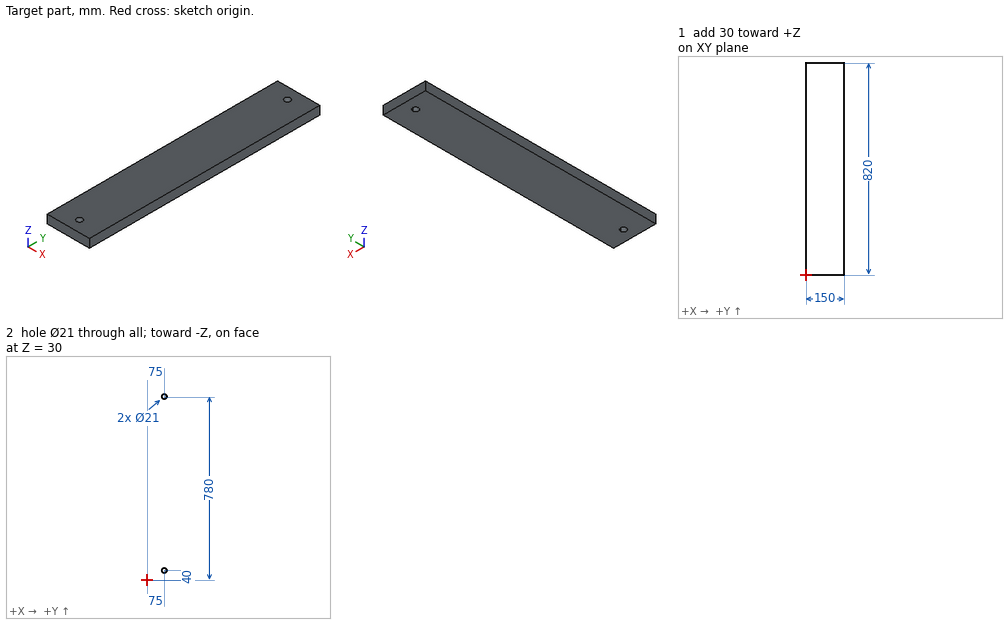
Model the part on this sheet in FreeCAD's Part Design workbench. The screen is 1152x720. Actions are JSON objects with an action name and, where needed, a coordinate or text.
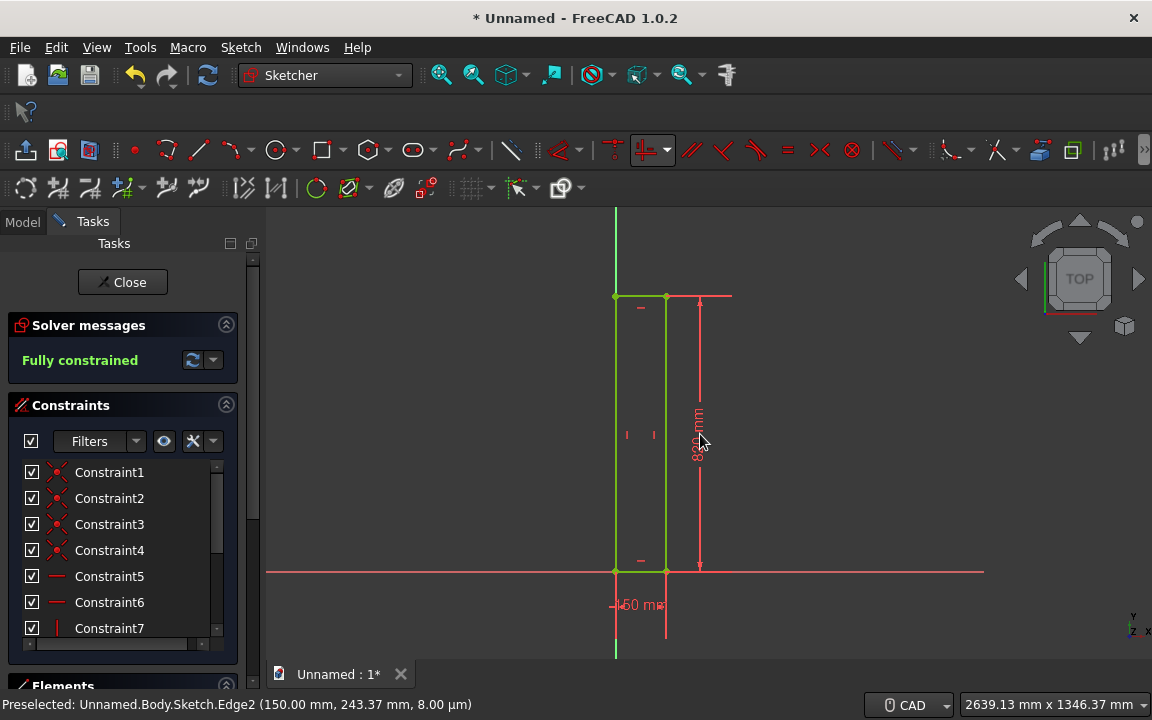
{"action": "left_click", "coordinate": [123, 282]}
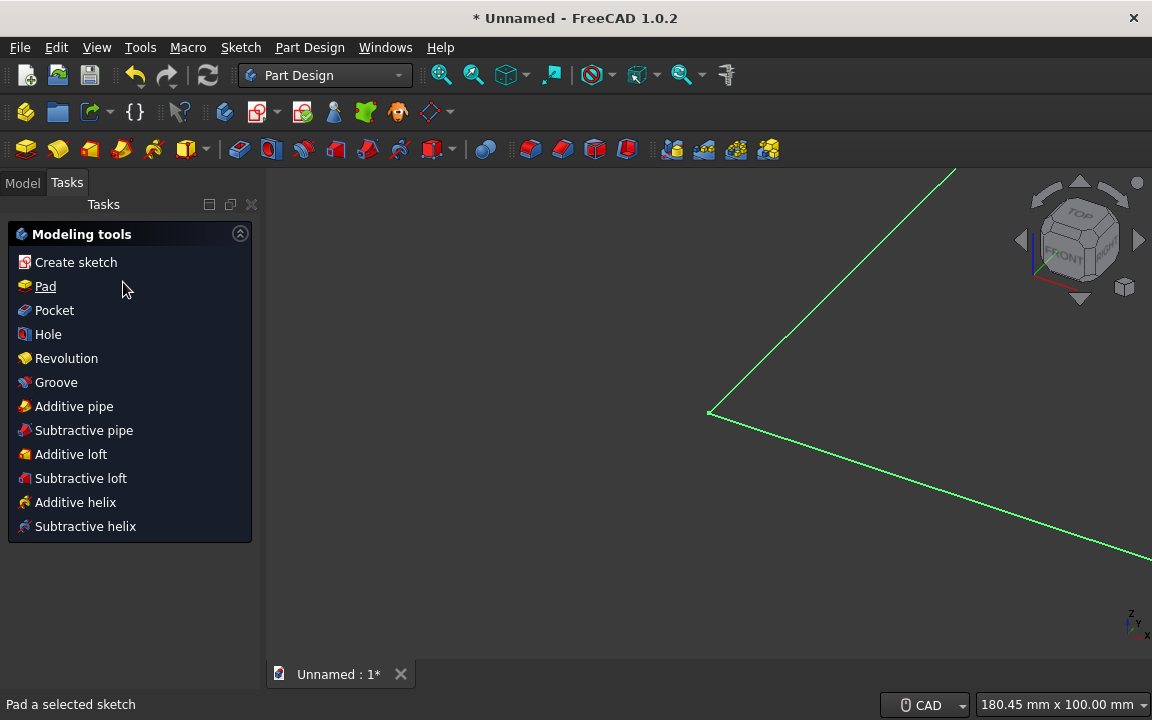
{"action": "left_click", "coordinate": [26, 150]}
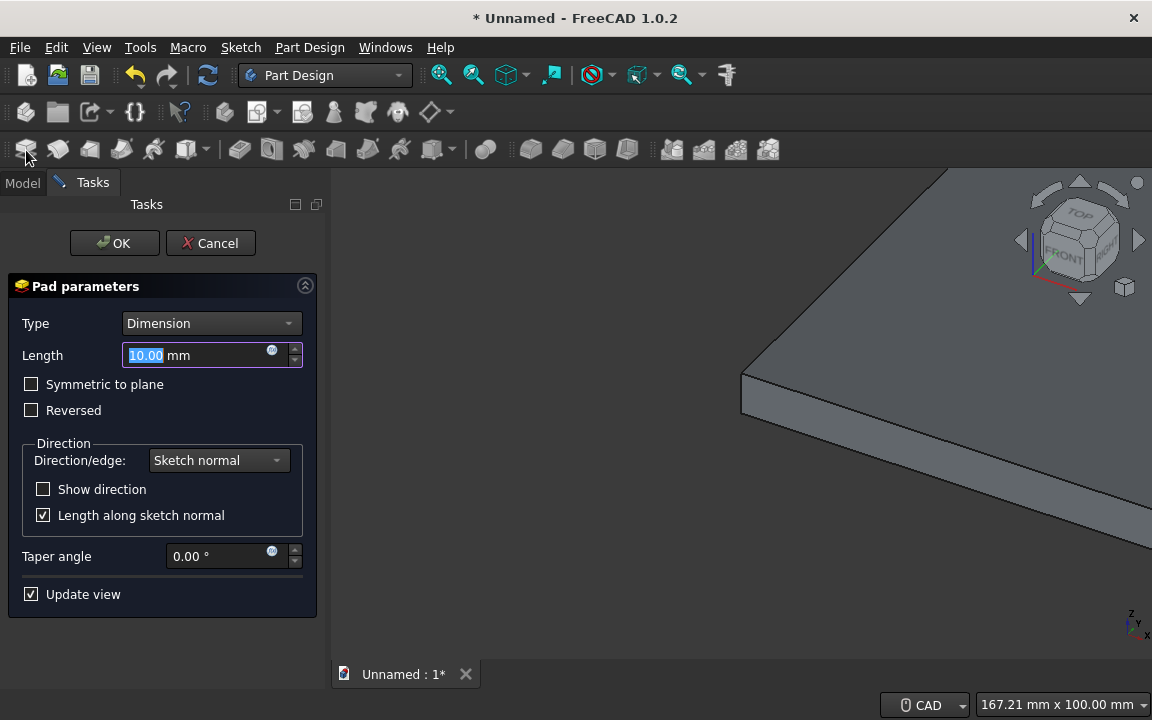
{"action": "type", "text": "30"}
{"action": "key", "text": "Tab"}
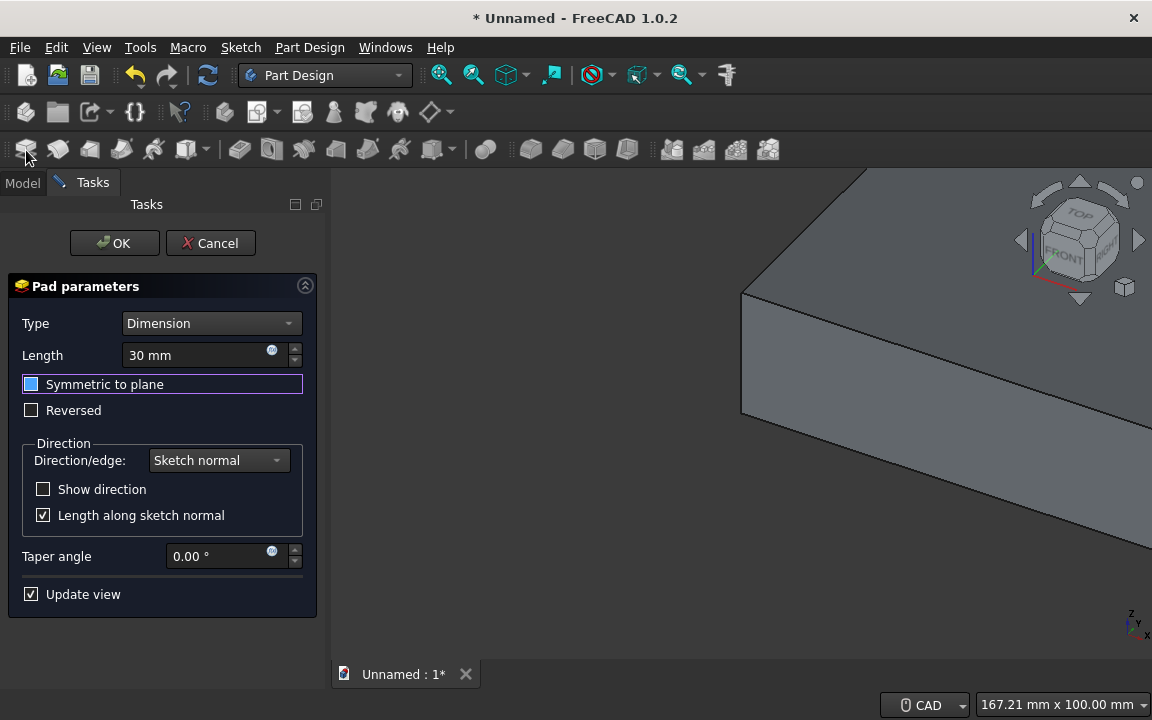
{"action": "left_click", "coordinate": [115, 243]}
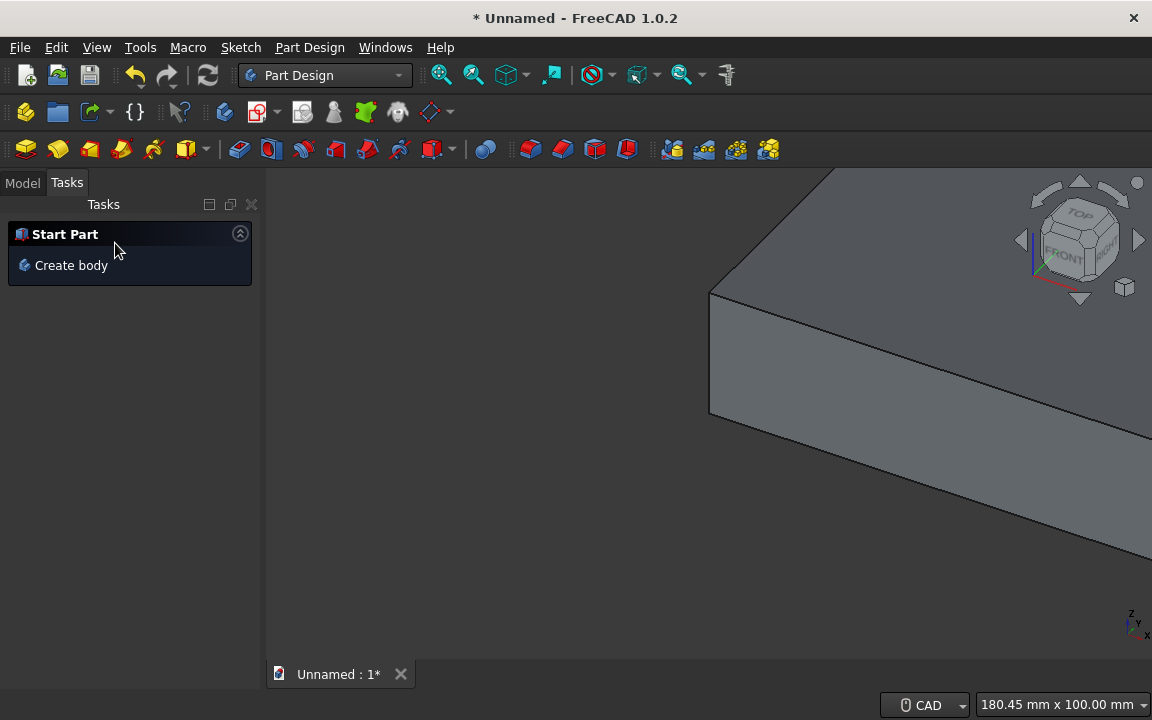
{"action": "left_click", "coordinate": [442, 76]}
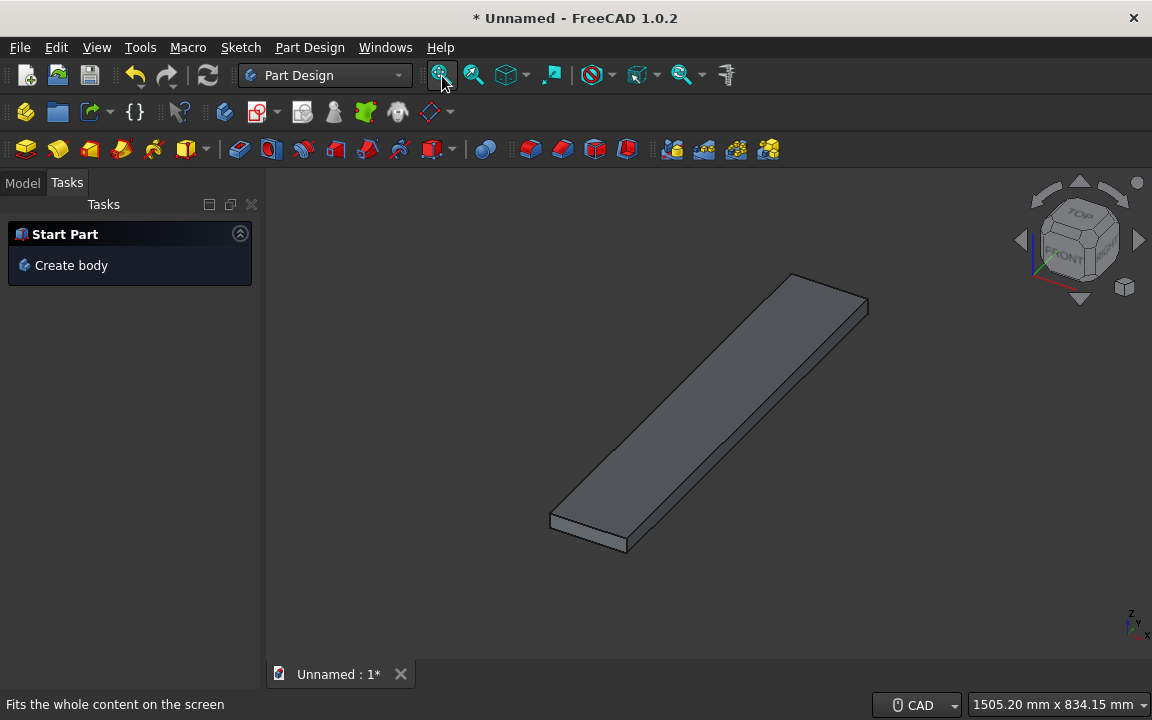
{"action": "left_click", "coordinate": [778, 337]}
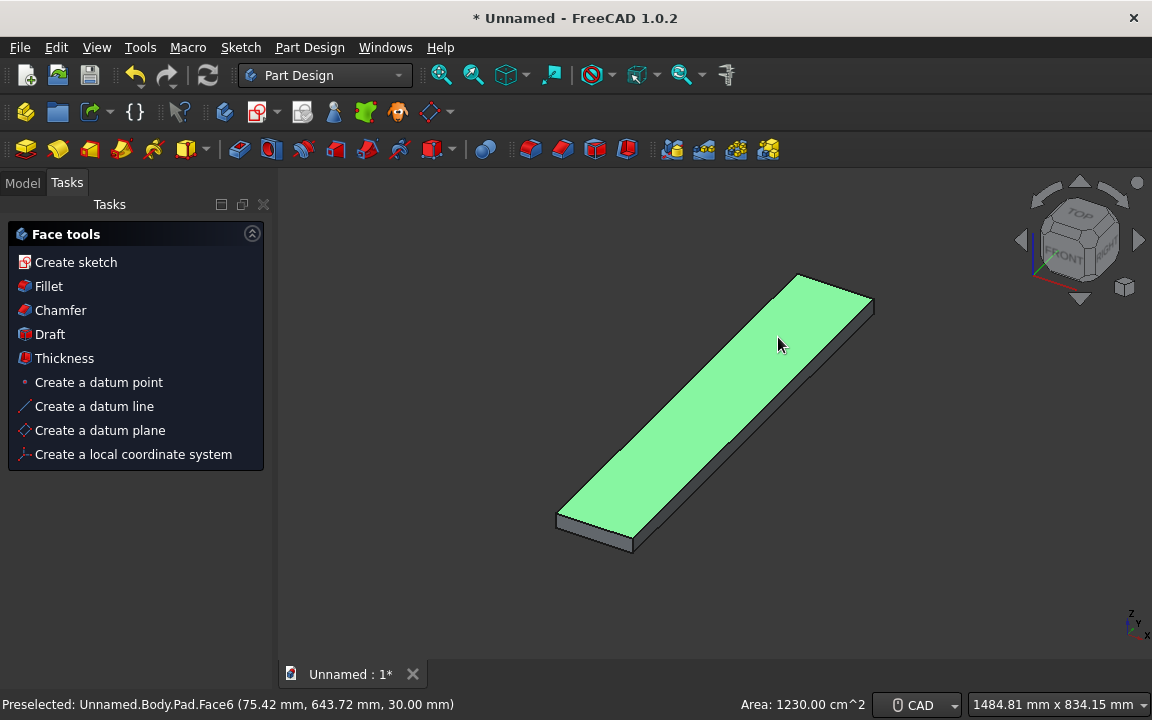
{"action": "left_click", "coordinate": [258, 112]}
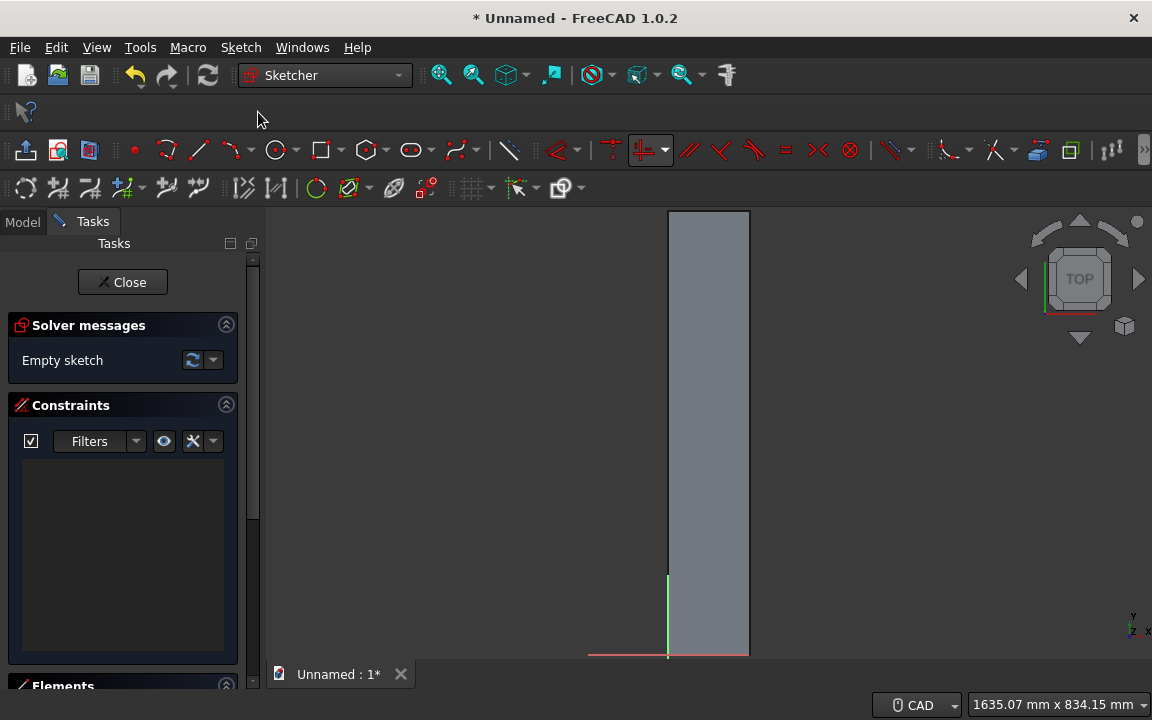
{"action": "scroll", "coordinate": [537, 417], "scroll_direction": "down", "scroll_amount": 2}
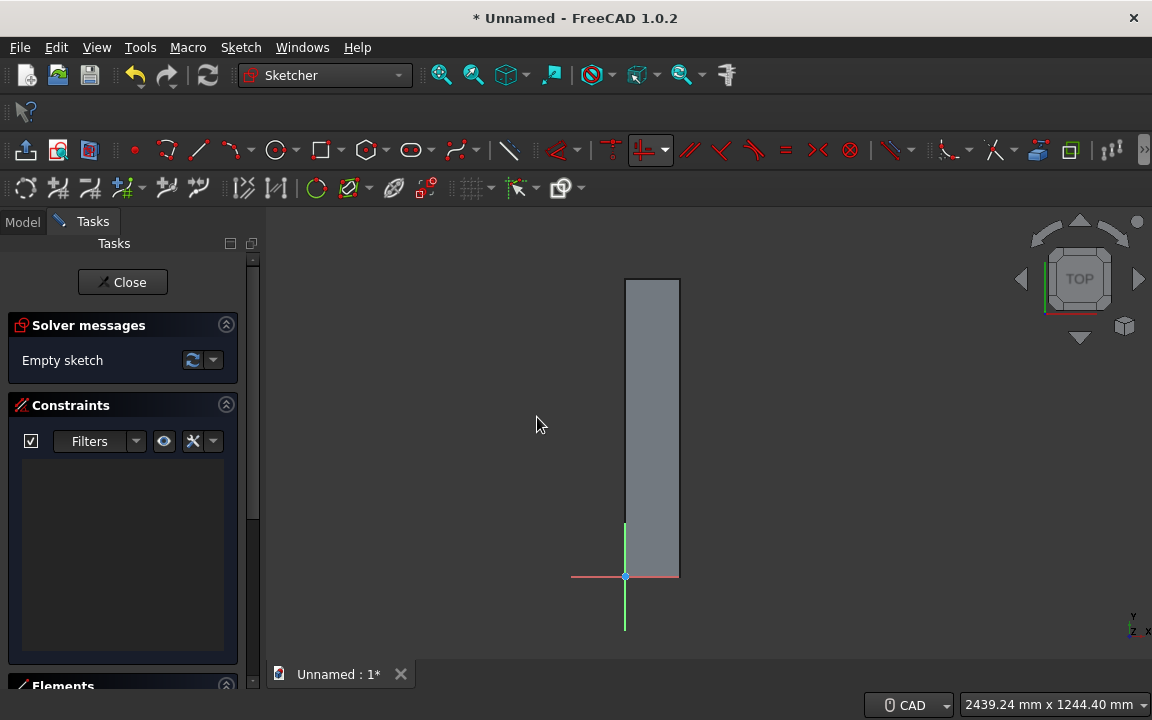
{"action": "left_click", "coordinate": [276, 150]}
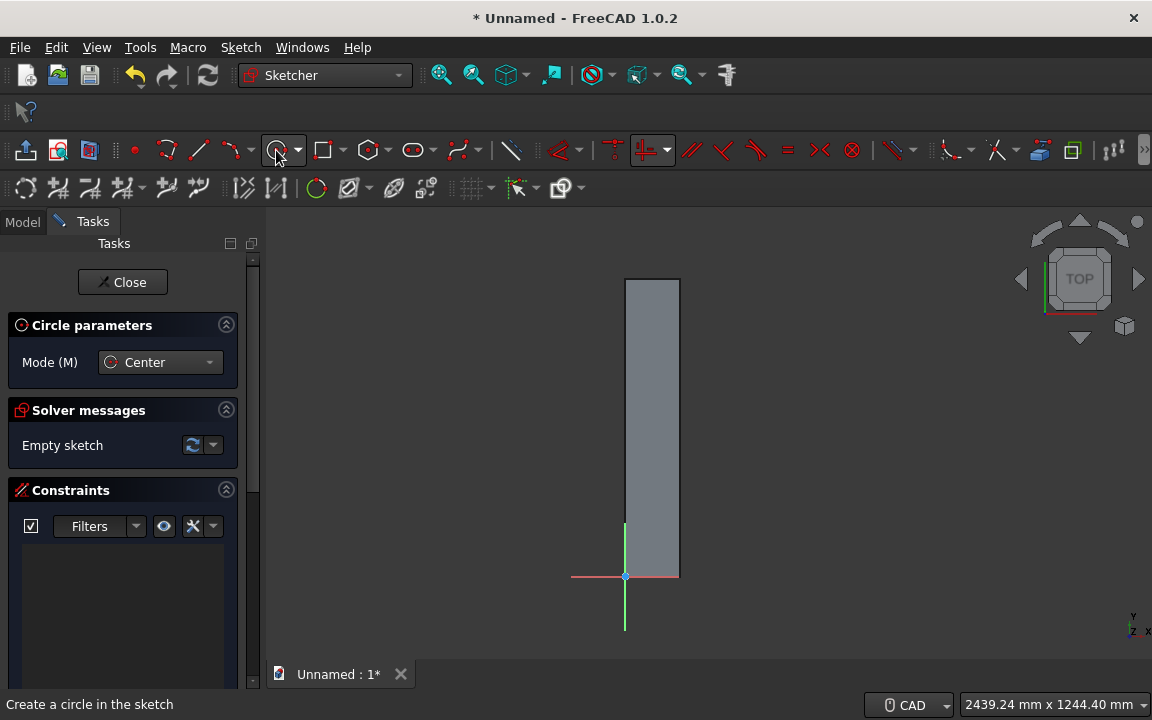
{"action": "scroll", "coordinate": [652, 293], "scroll_direction": "up", "scroll_amount": 9}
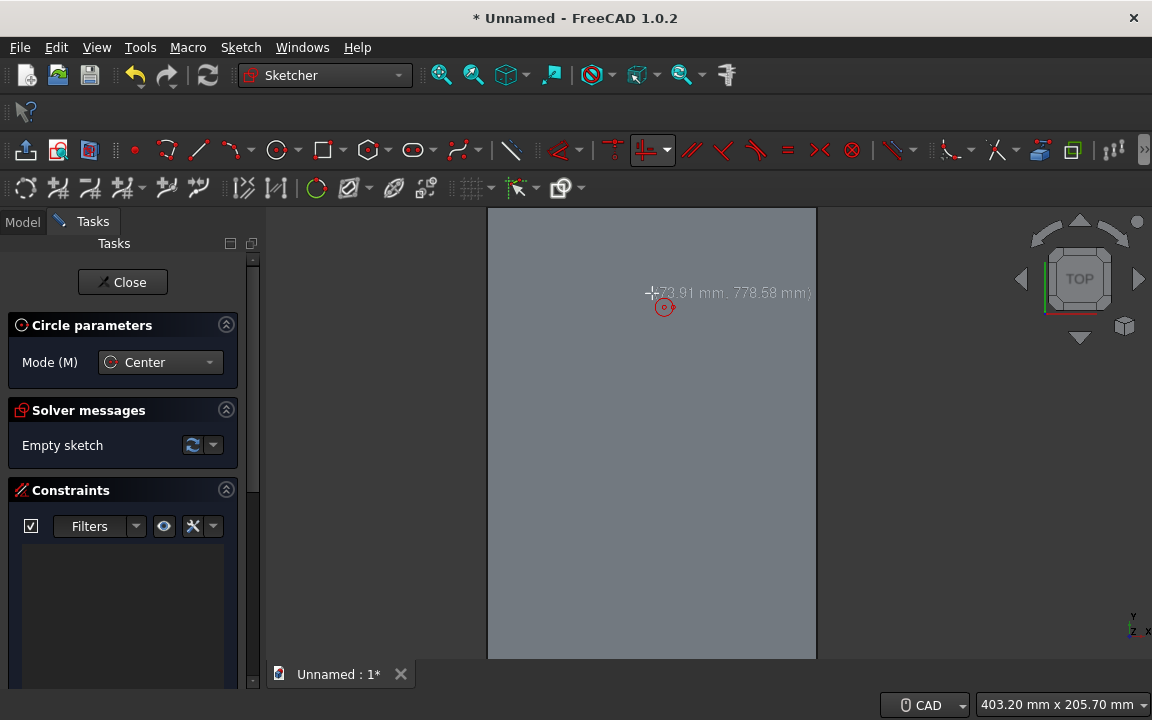
{"action": "scroll", "coordinate": [652, 293], "scroll_direction": "down", "scroll_amount": 9}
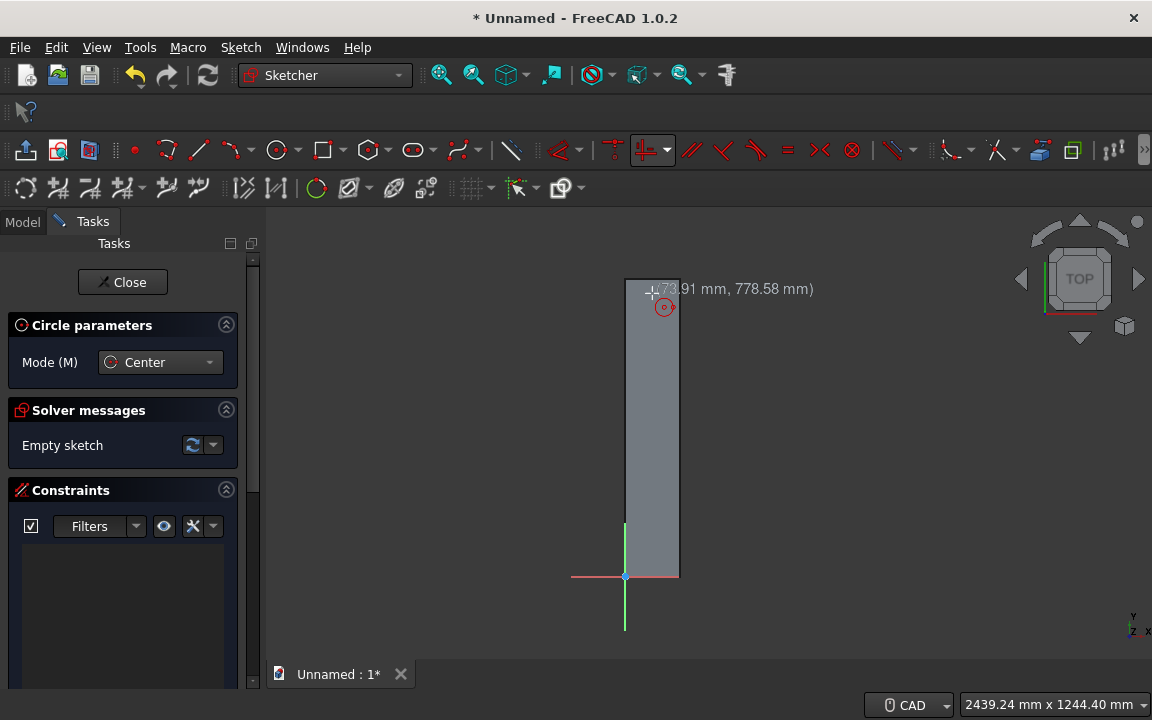
{"action": "left_click", "coordinate": [652, 293]}